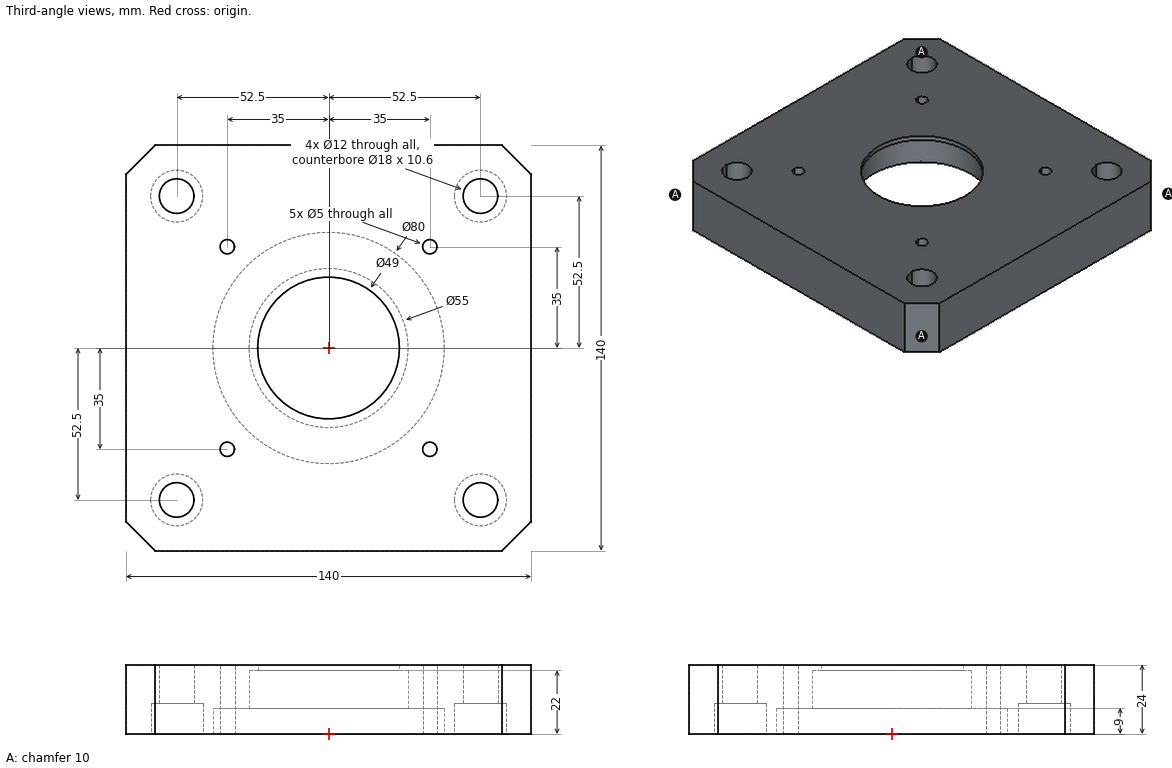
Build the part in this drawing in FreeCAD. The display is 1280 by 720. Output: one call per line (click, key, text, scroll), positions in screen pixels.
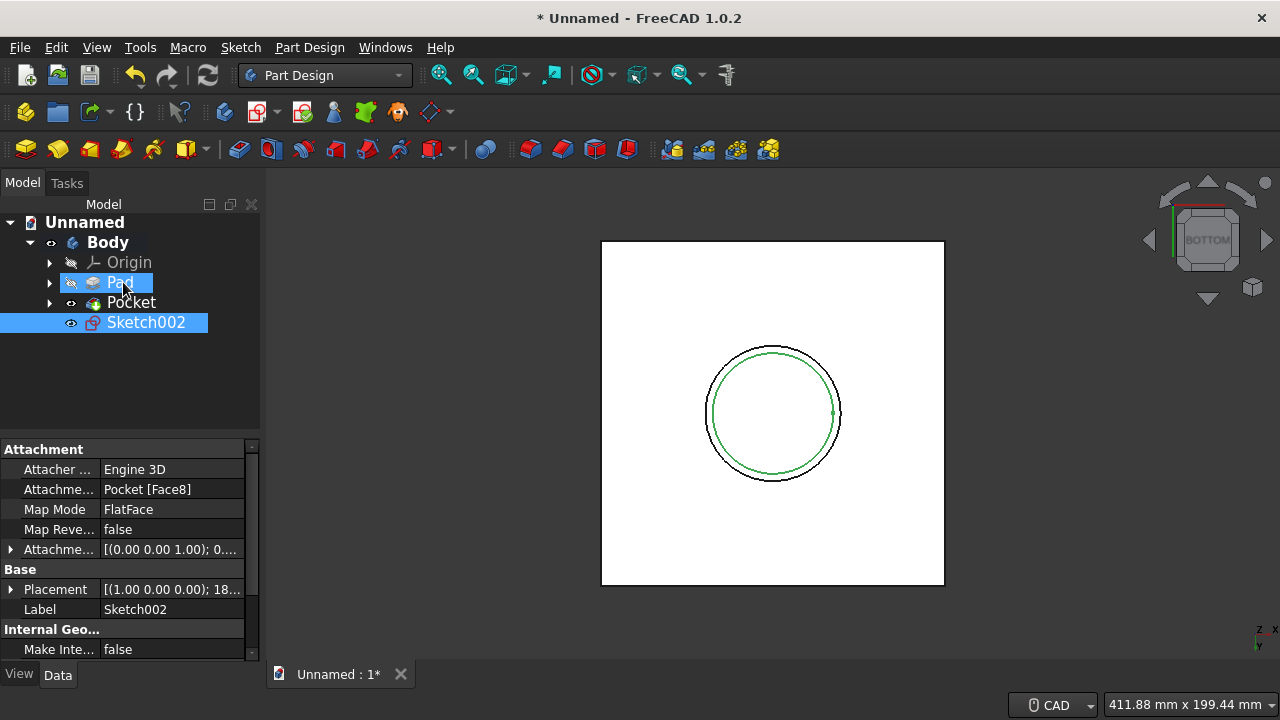
click(240, 150)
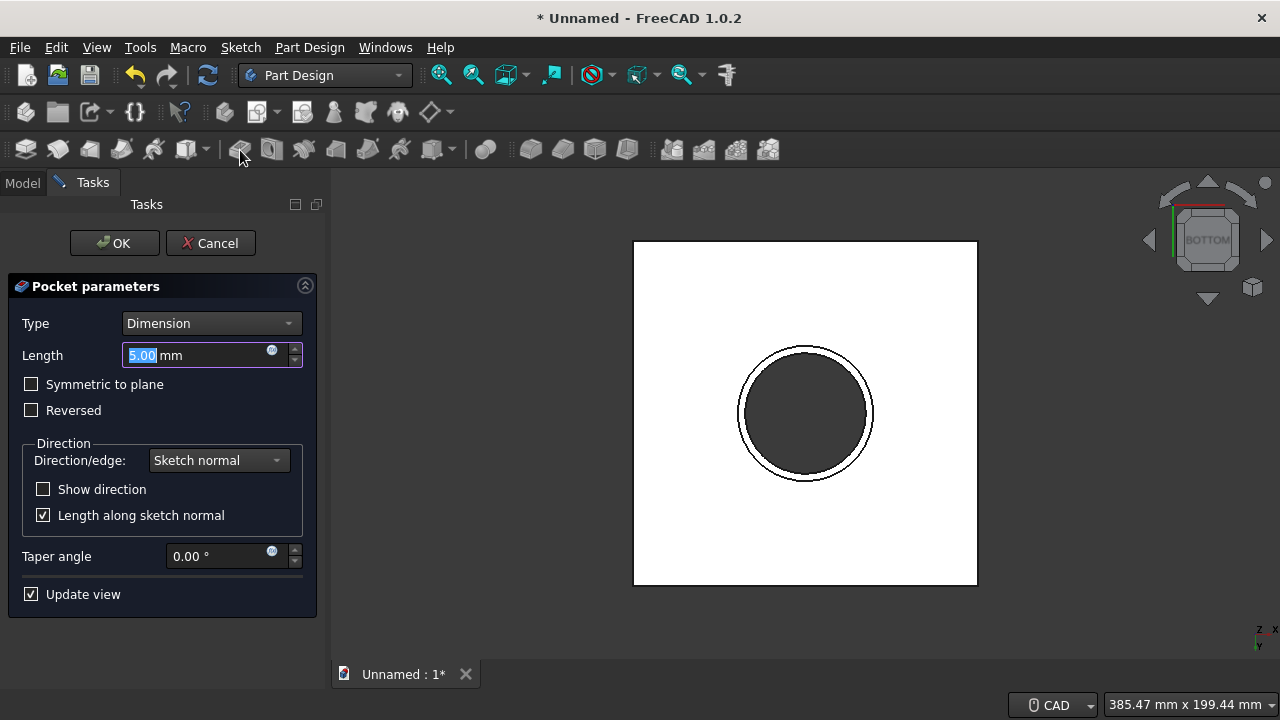
click(212, 324)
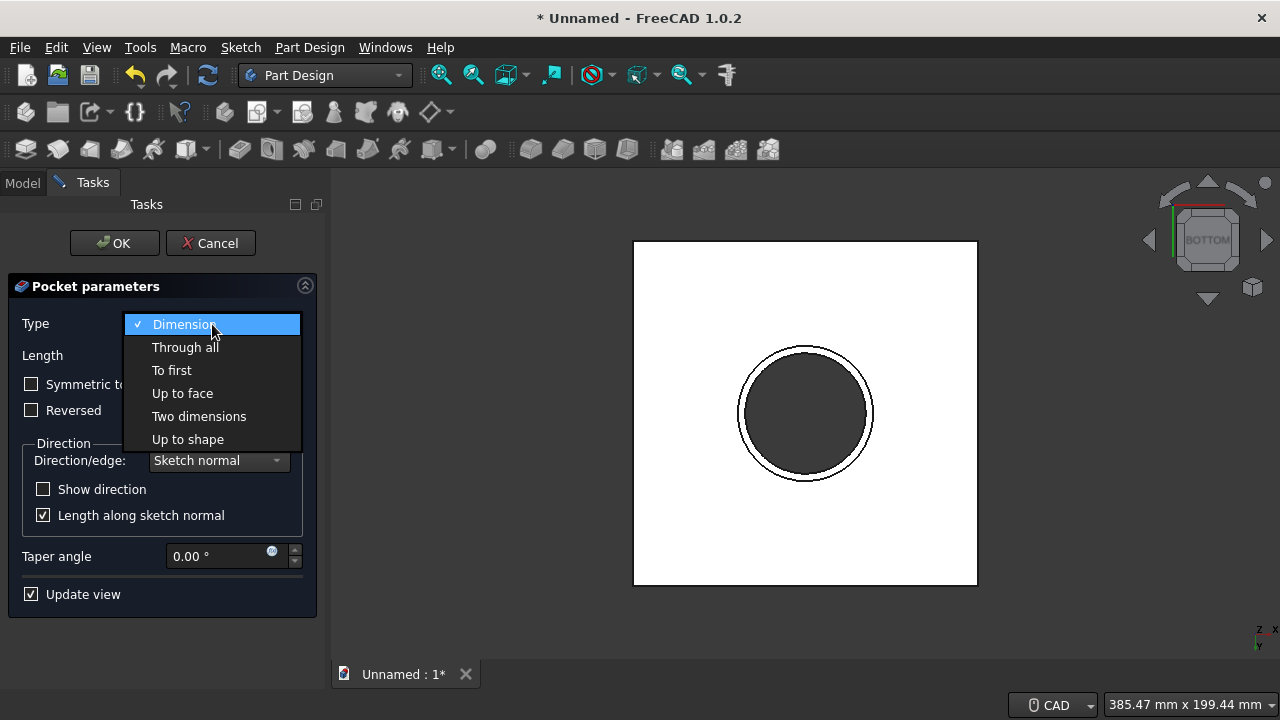
click(212, 348)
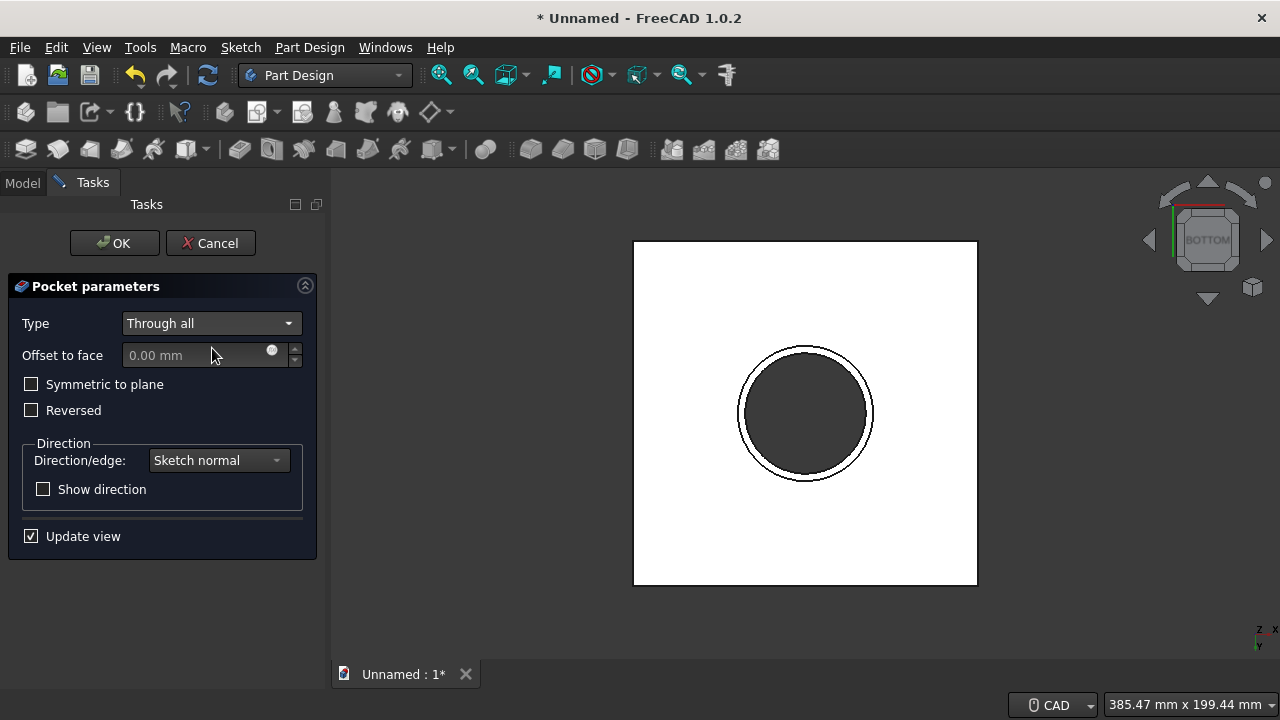
click(115, 243)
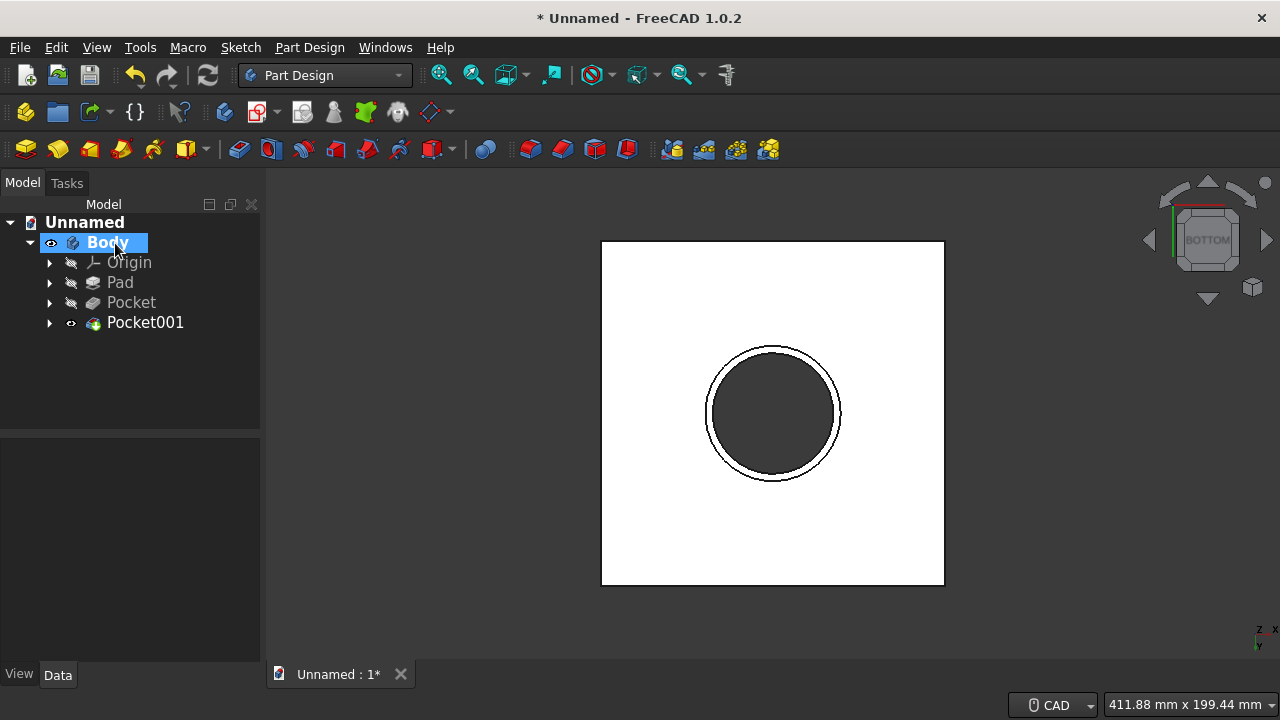
click(871, 511)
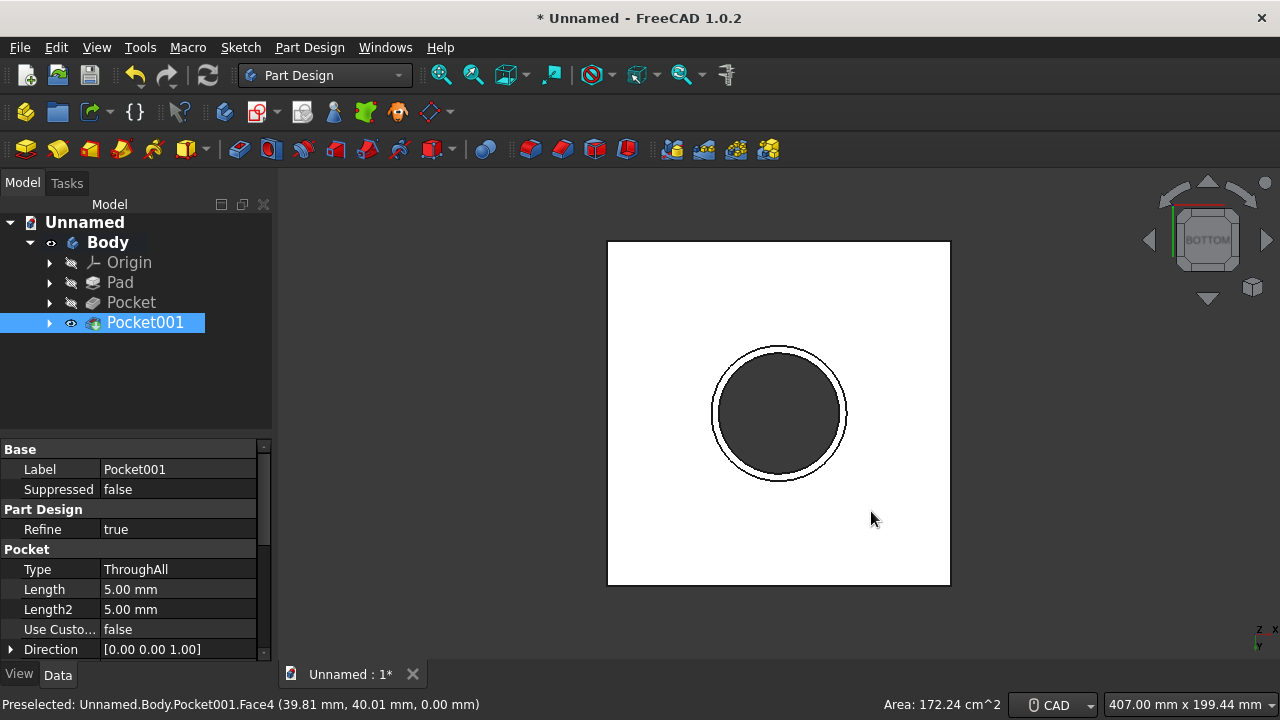
click(258, 112)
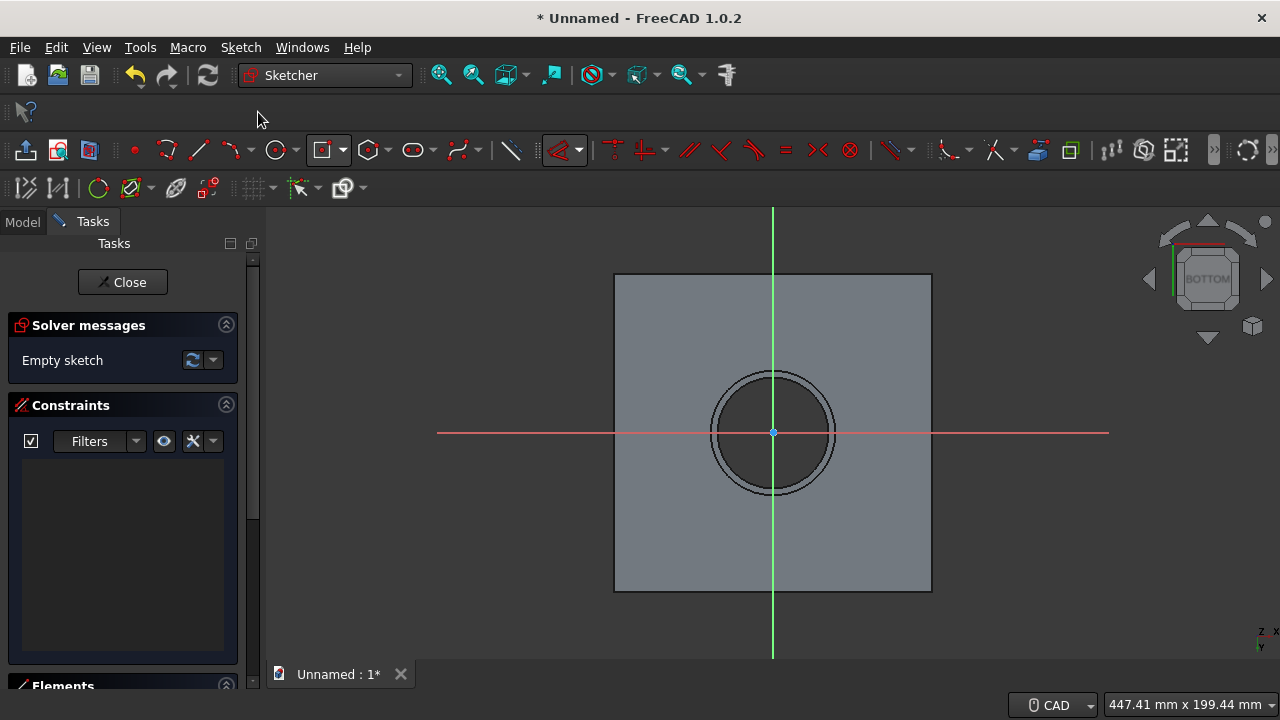
click(276, 150)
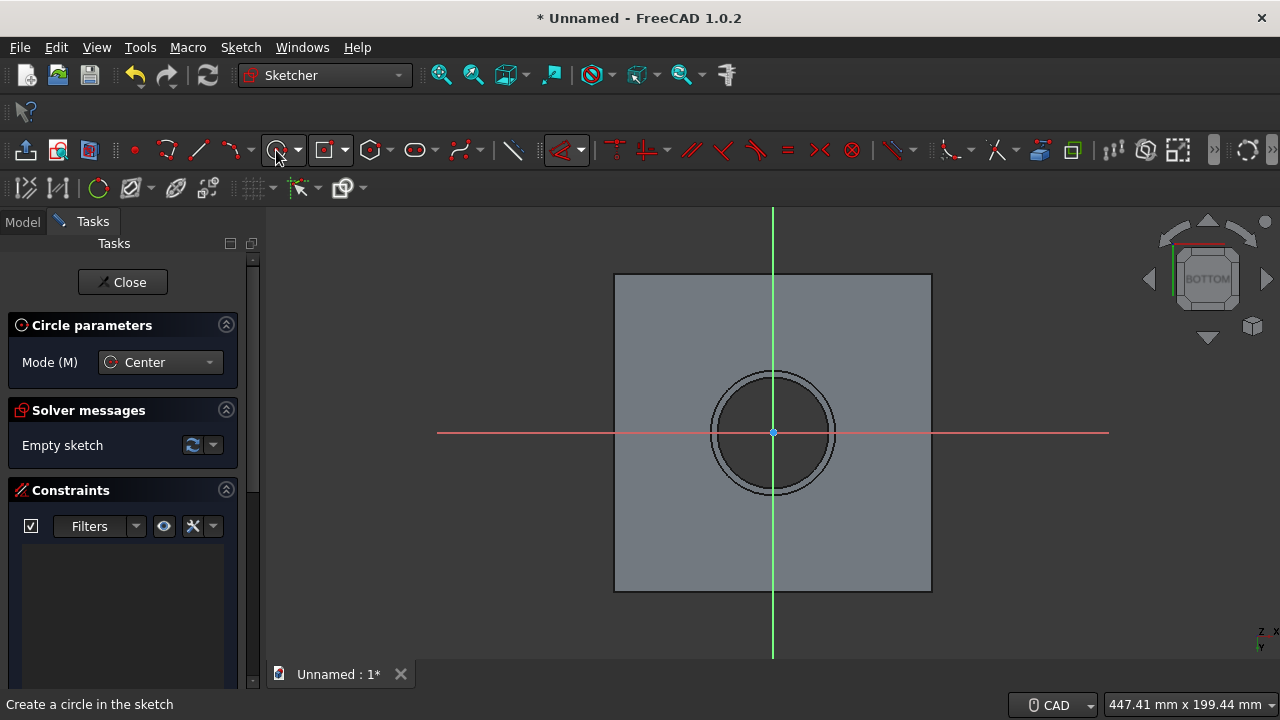
scroll(892, 552, up, 3)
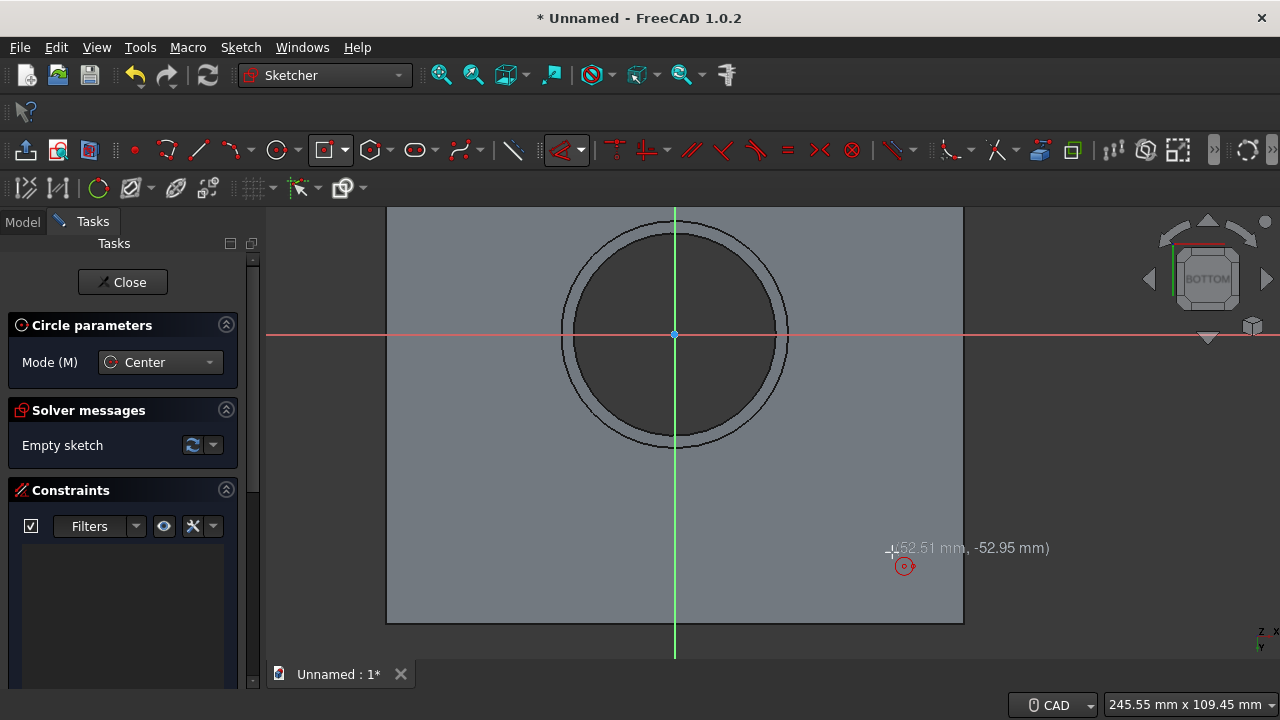
click(891, 551)
move(909, 534)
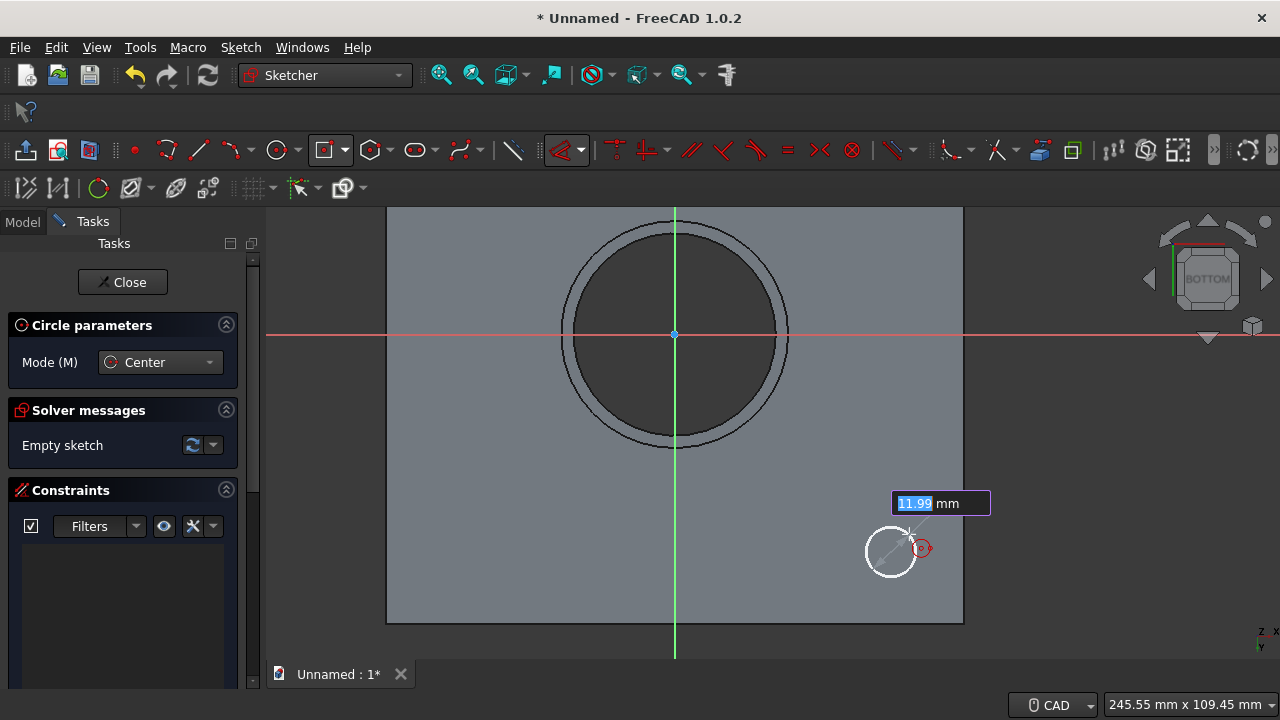
text(12)
key(Return)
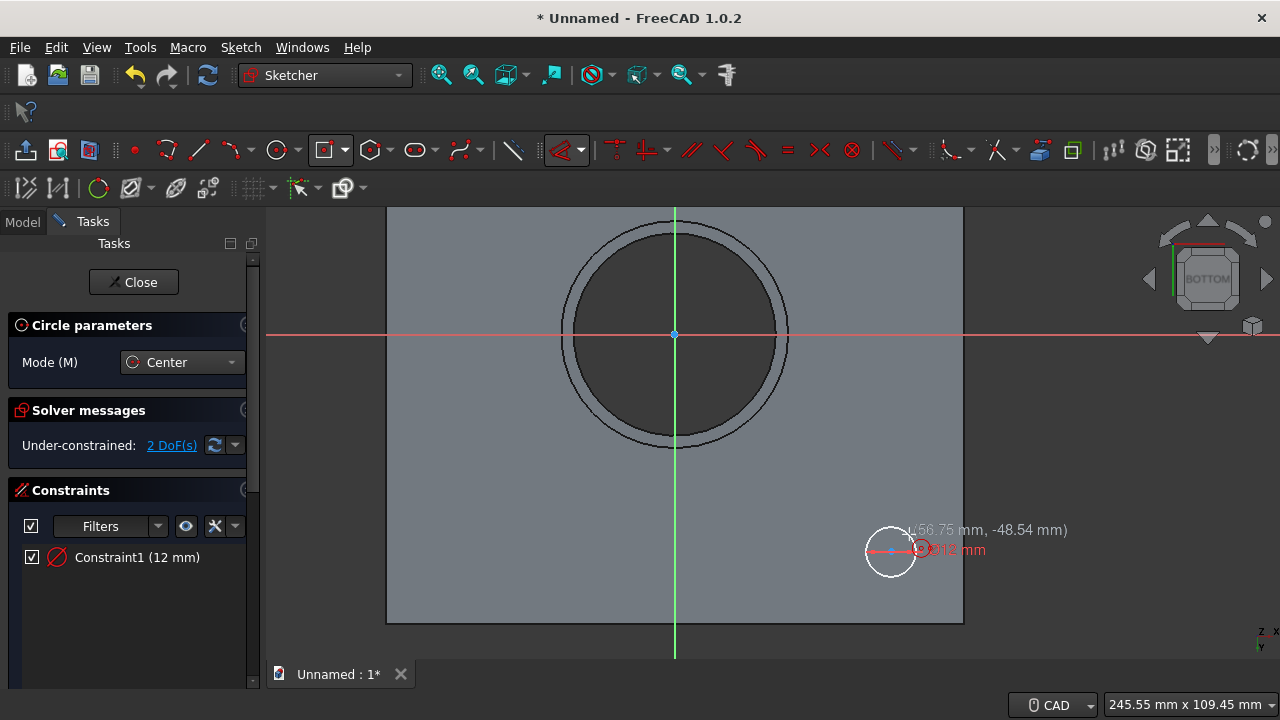
click(458, 551)
move(475, 534)